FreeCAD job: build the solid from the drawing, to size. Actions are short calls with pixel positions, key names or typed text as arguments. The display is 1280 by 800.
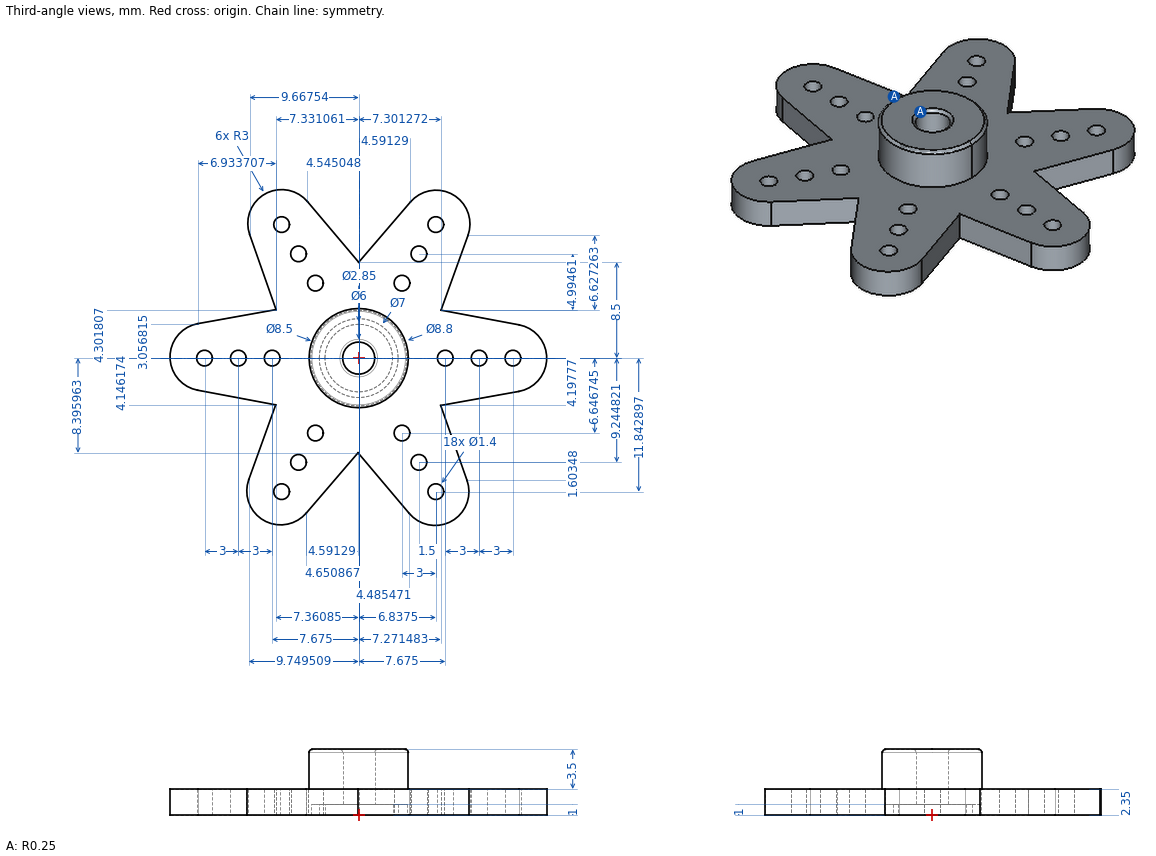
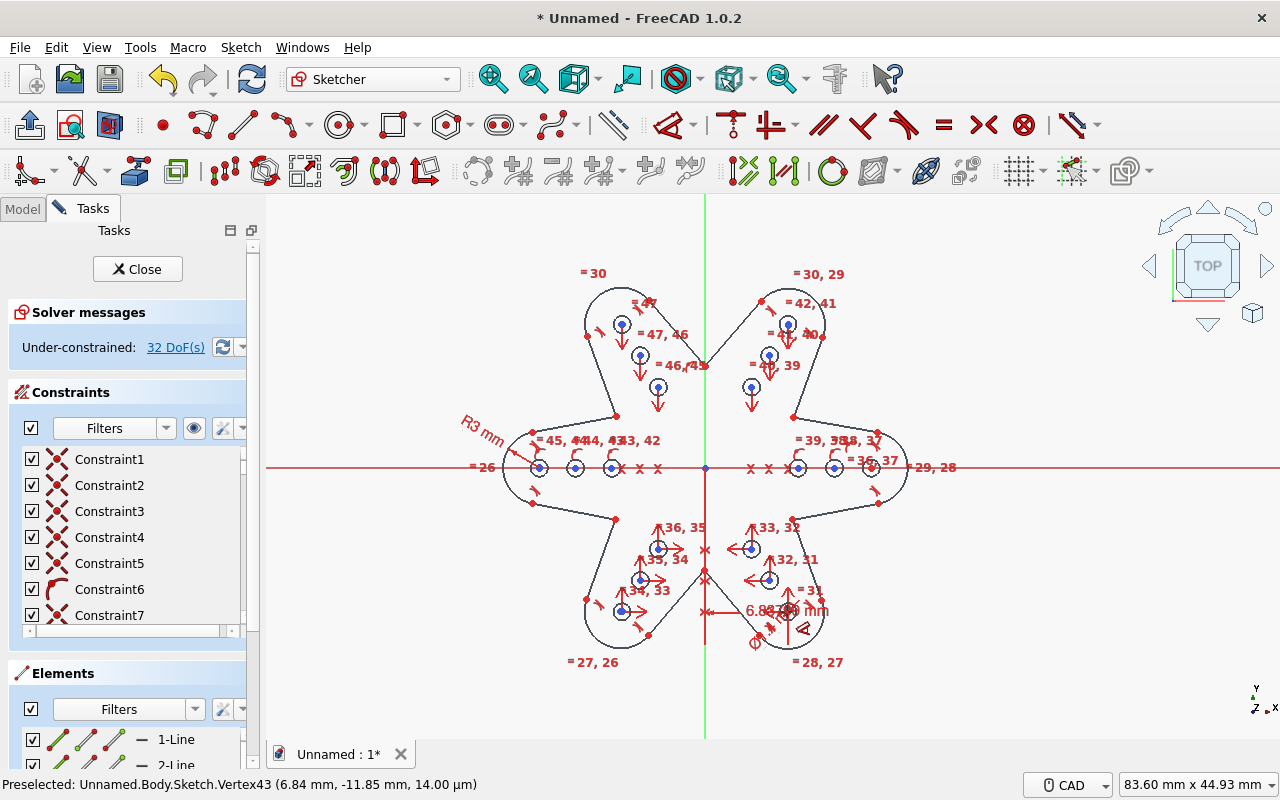
click(752, 549)
click(770, 515)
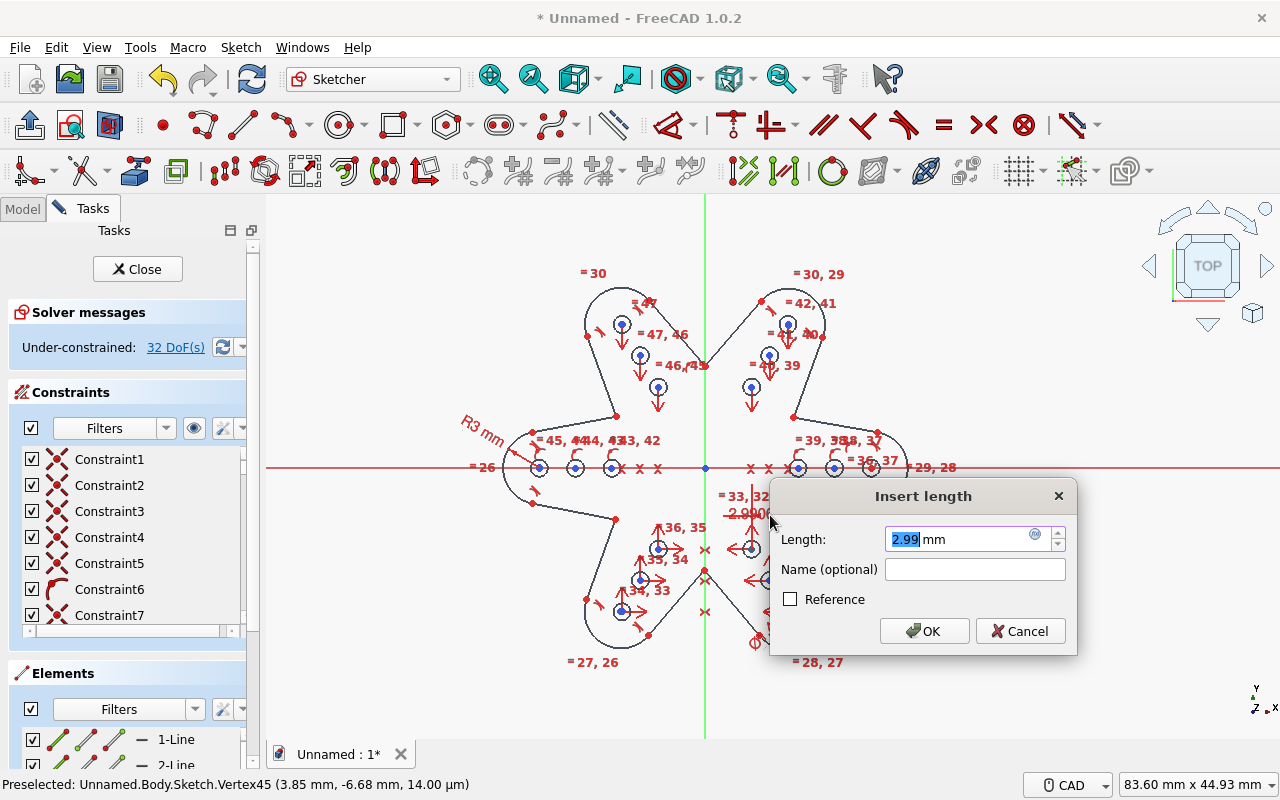
text(3)
key(Return)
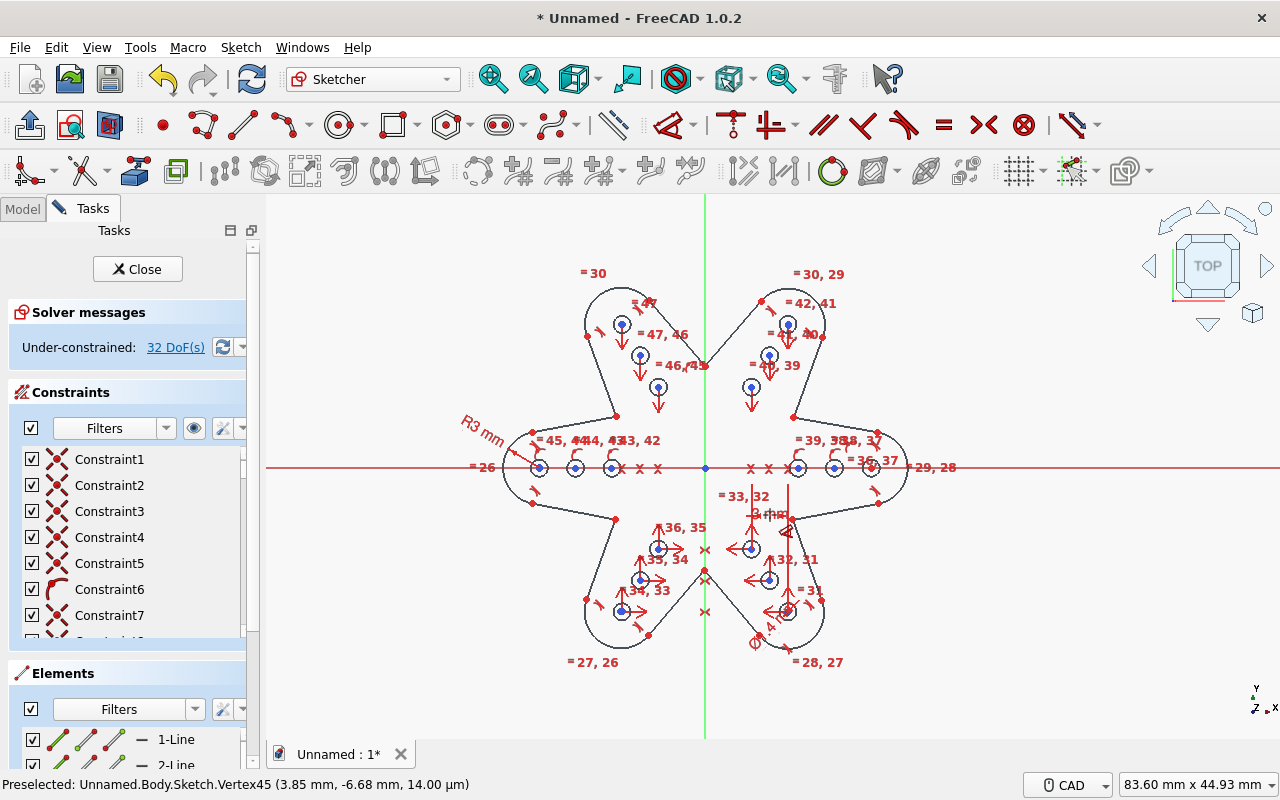
click(871, 468)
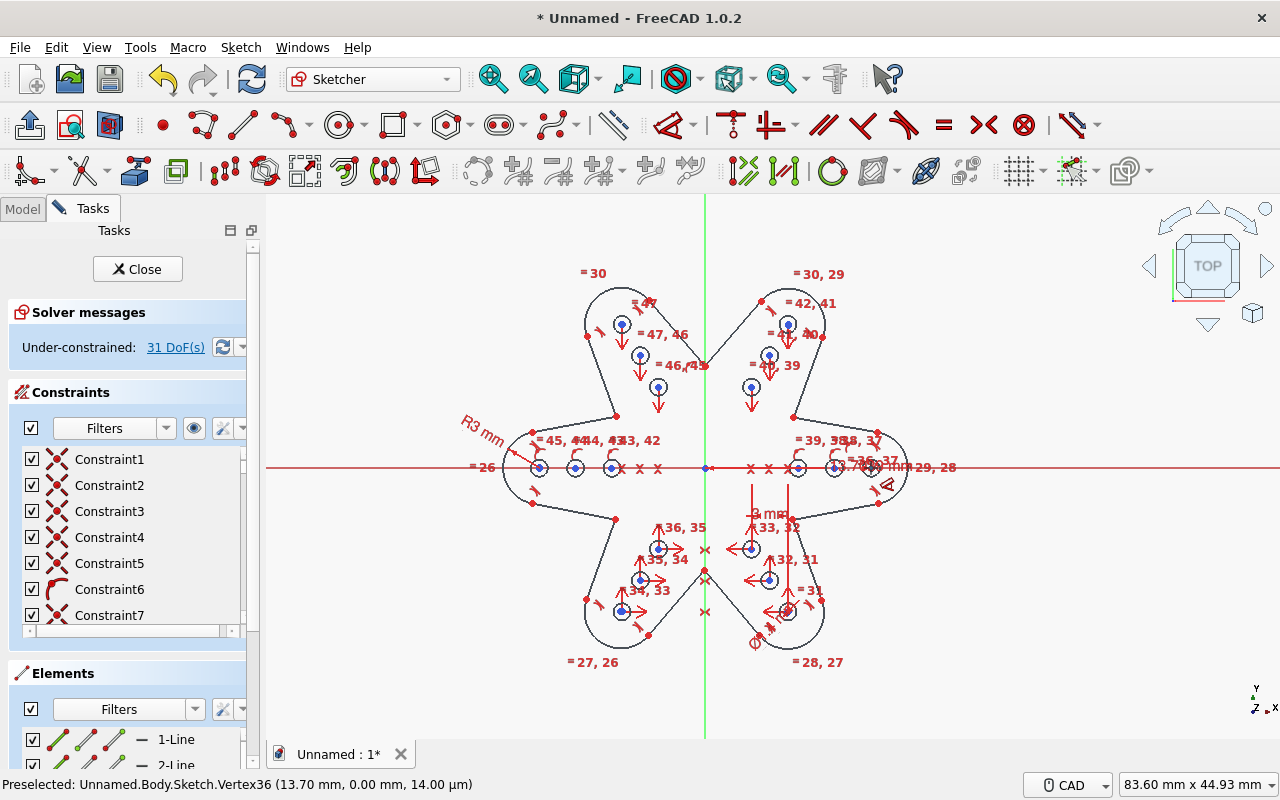
click(835, 468)
click(853, 526)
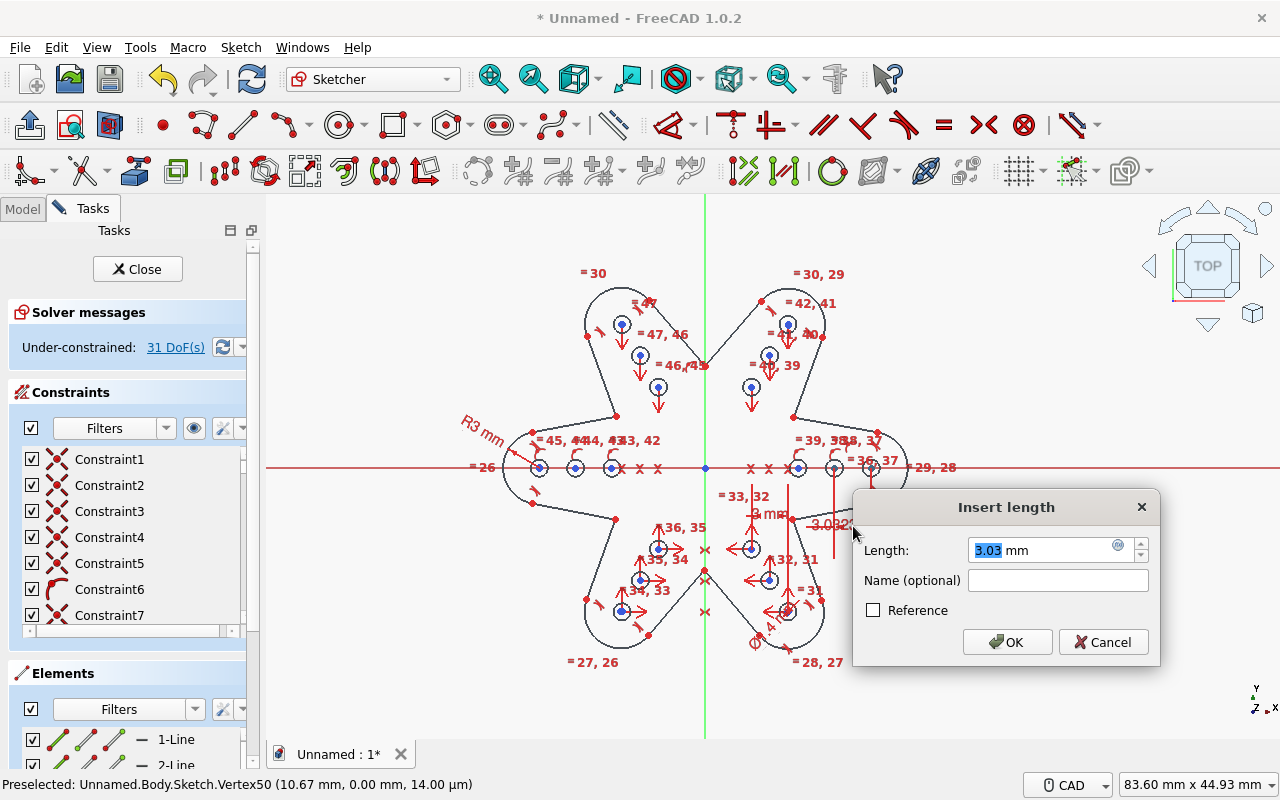
text(3)
key(Return)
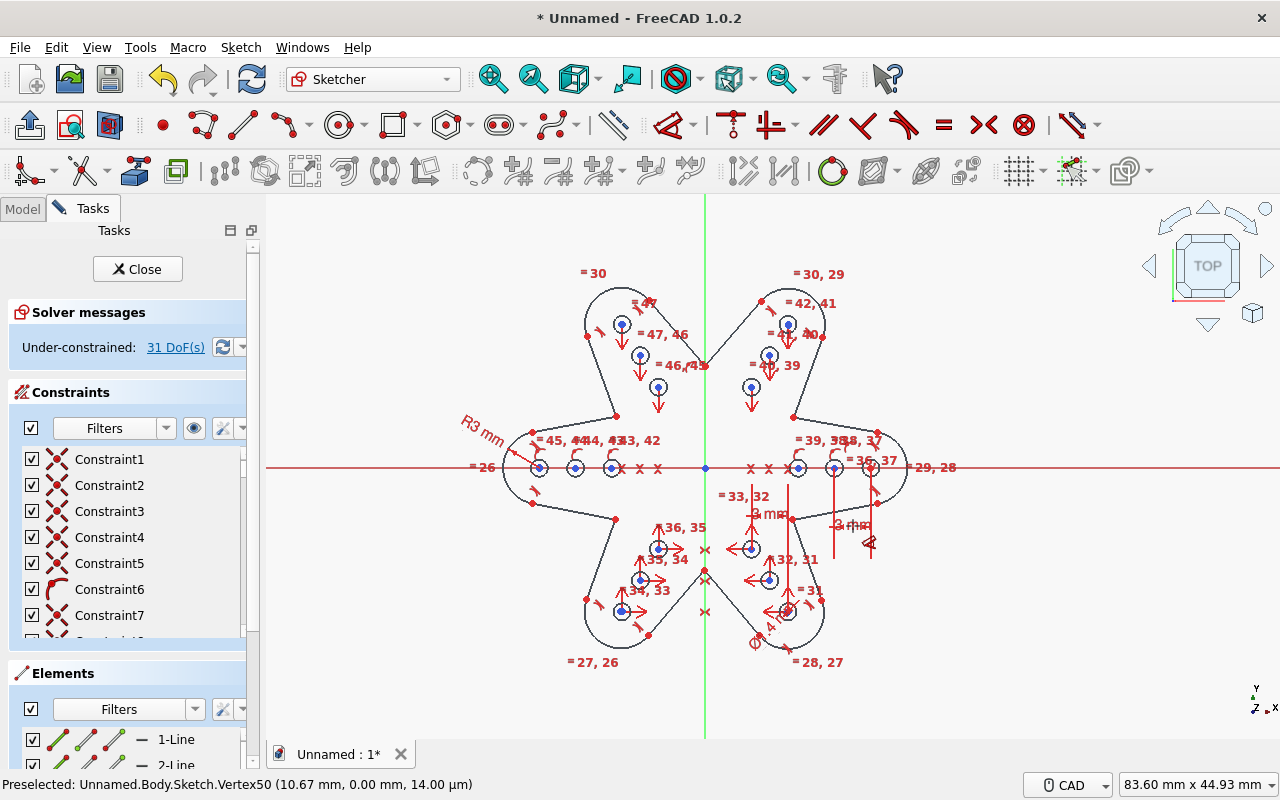
click(835, 468)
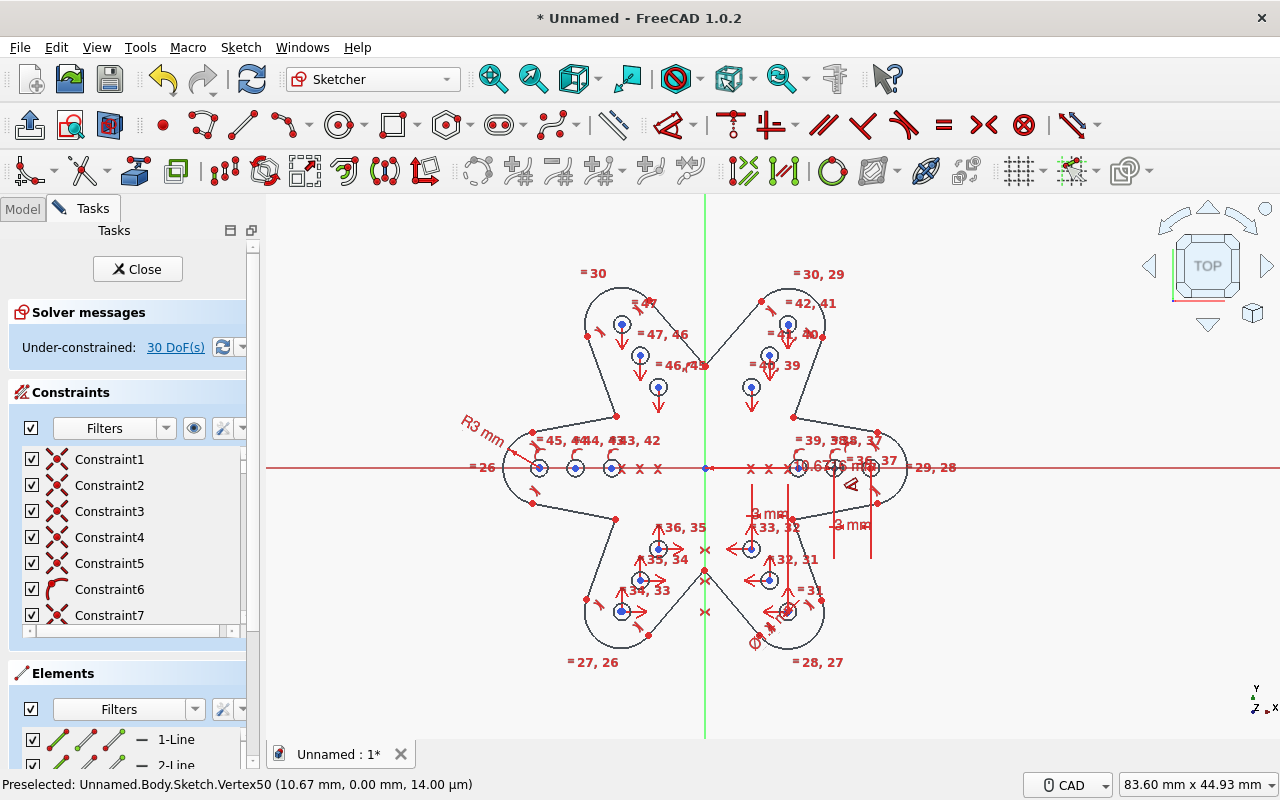
click(798, 468)
click(808, 434)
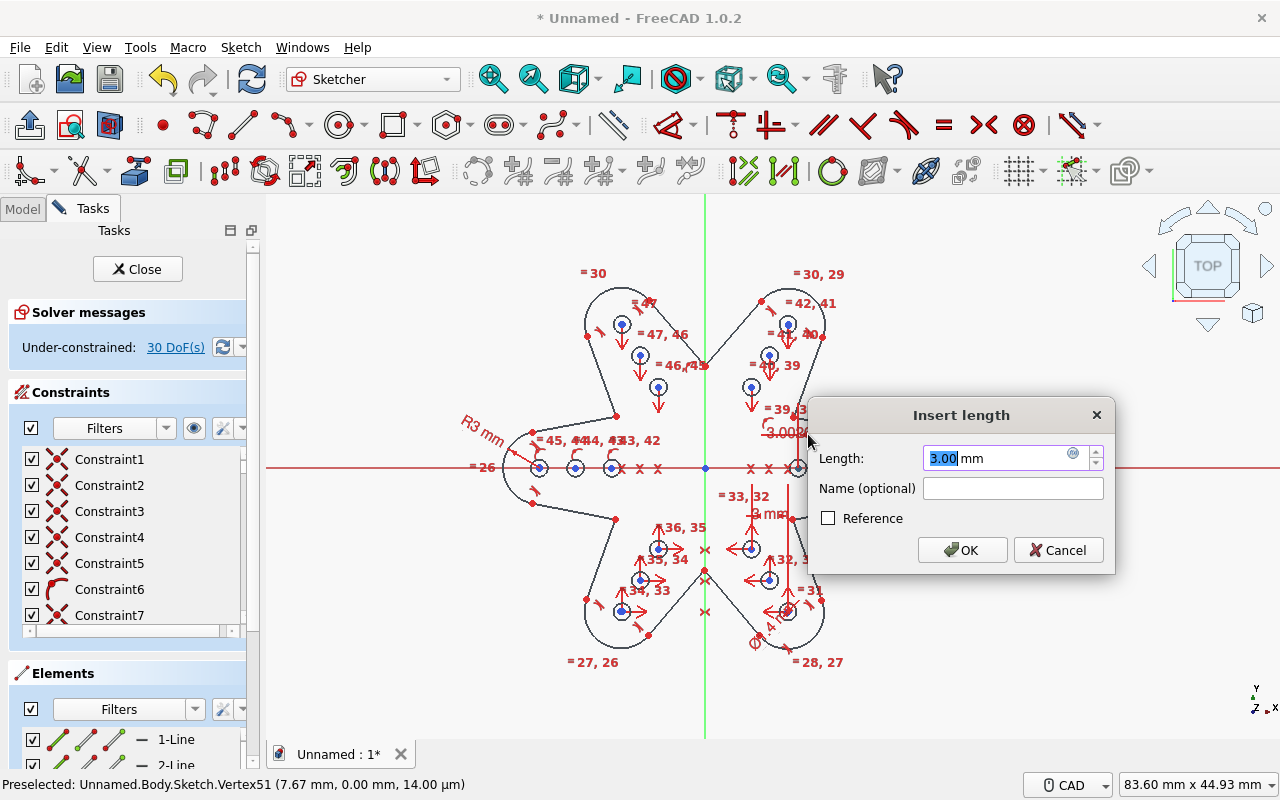
text(3)
key(Return)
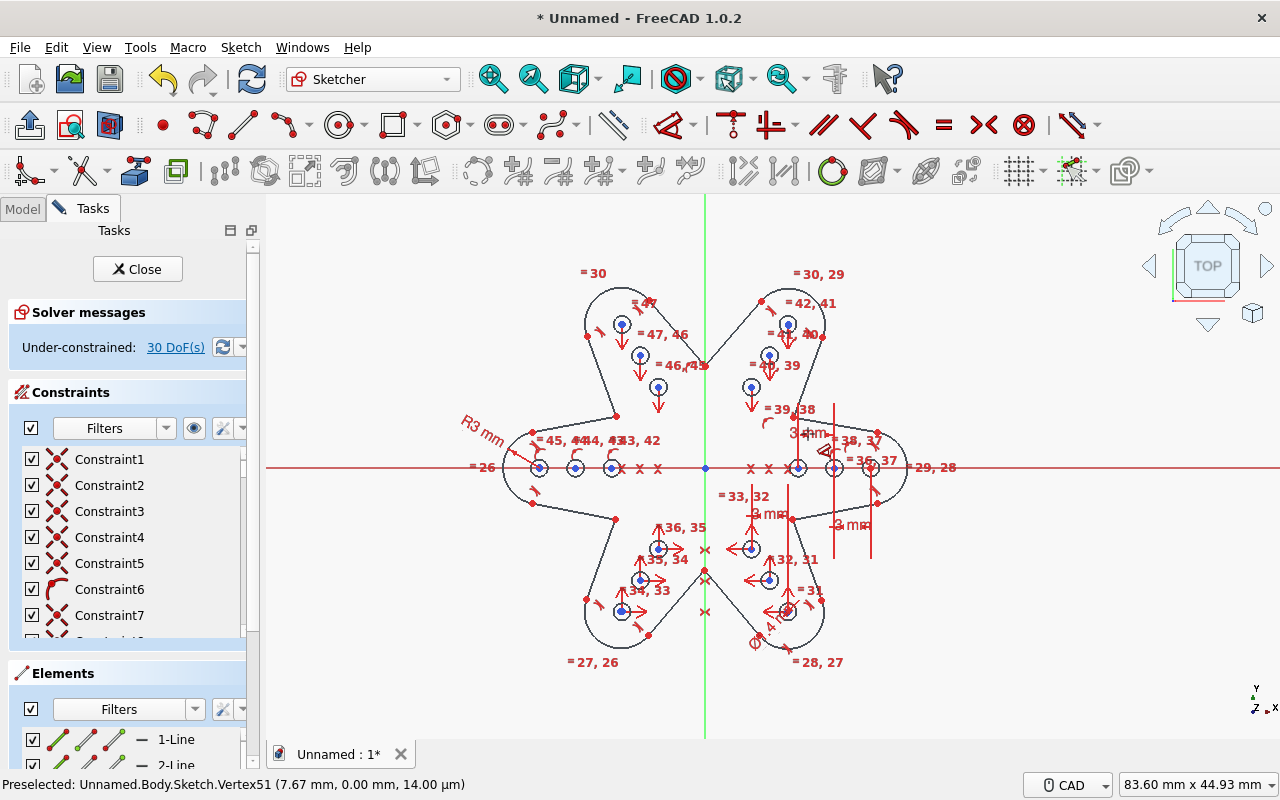
click(612, 468)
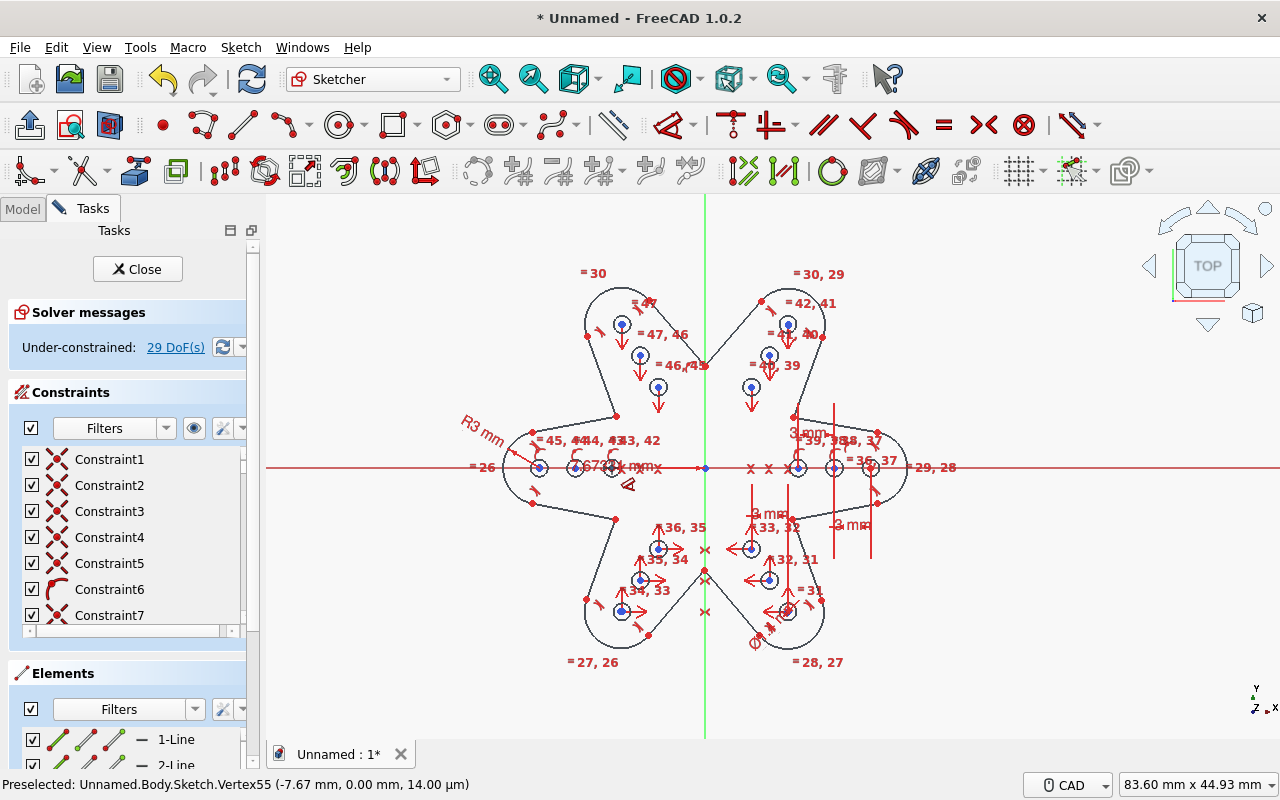
click(576, 468)
click(594, 502)